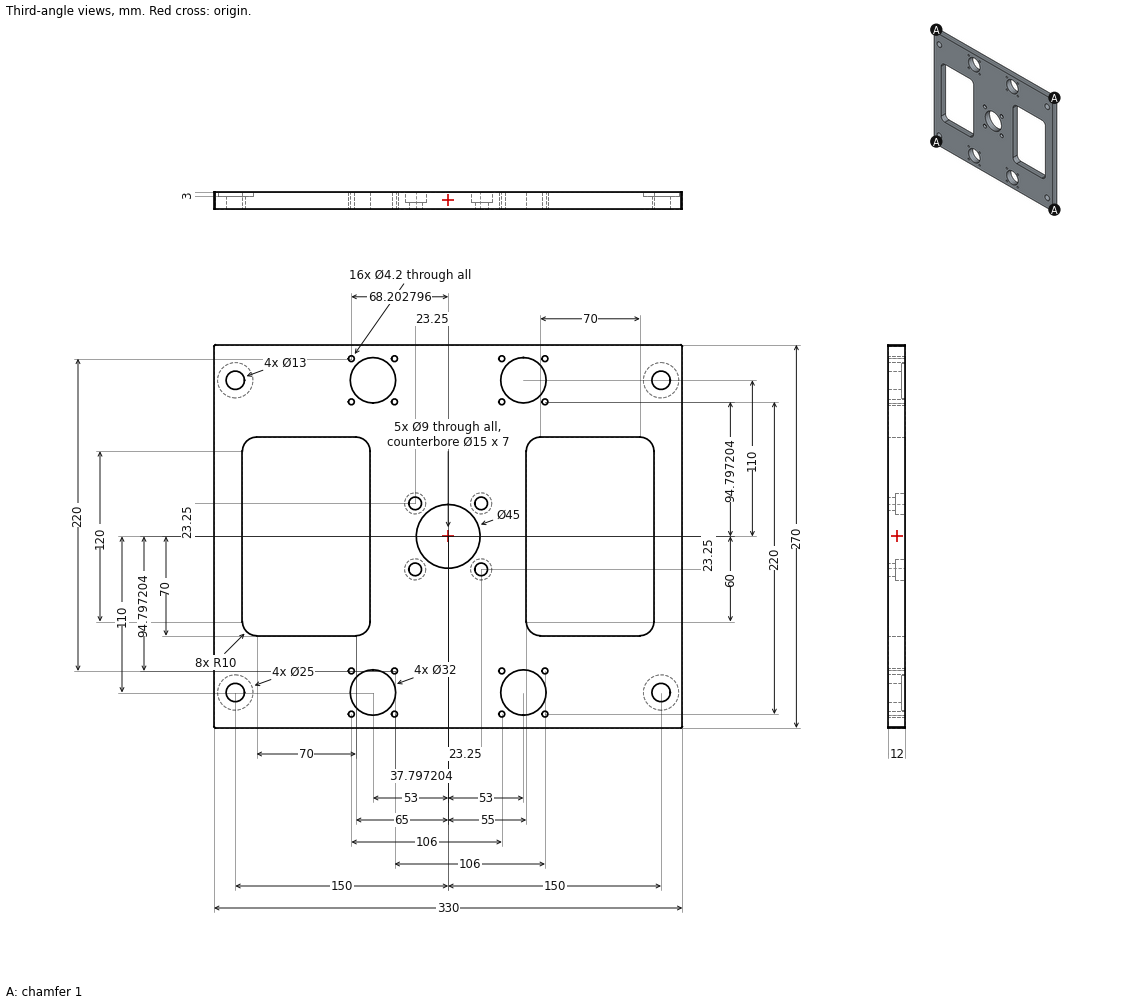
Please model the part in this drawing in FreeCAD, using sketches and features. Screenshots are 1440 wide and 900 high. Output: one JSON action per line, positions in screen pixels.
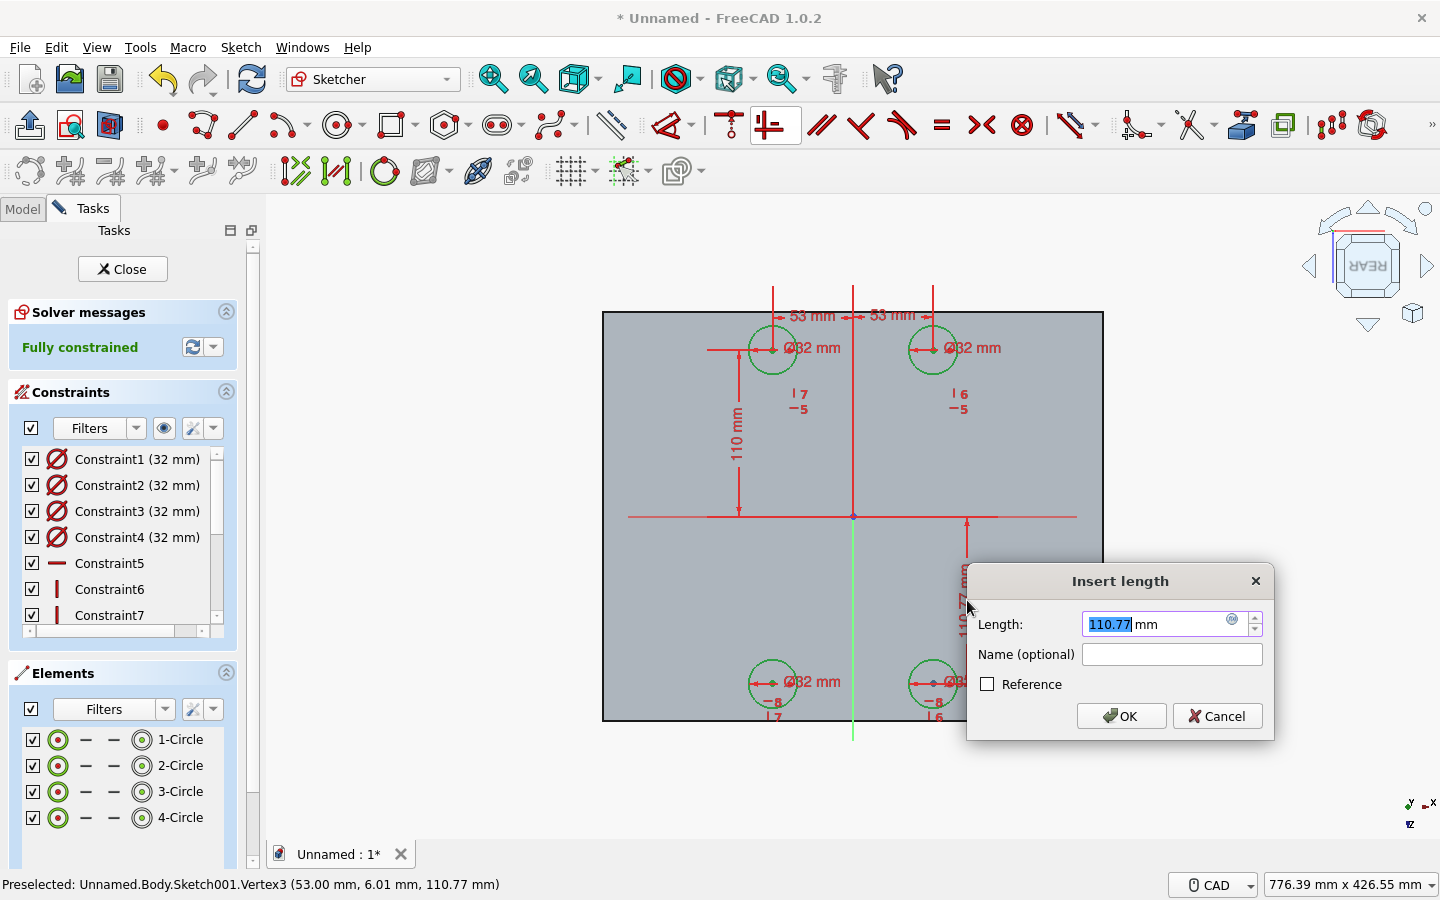
{"action": "type", "text": "110"}
{"action": "key", "text": "Return"}
{"action": "key", "text": "Escape"}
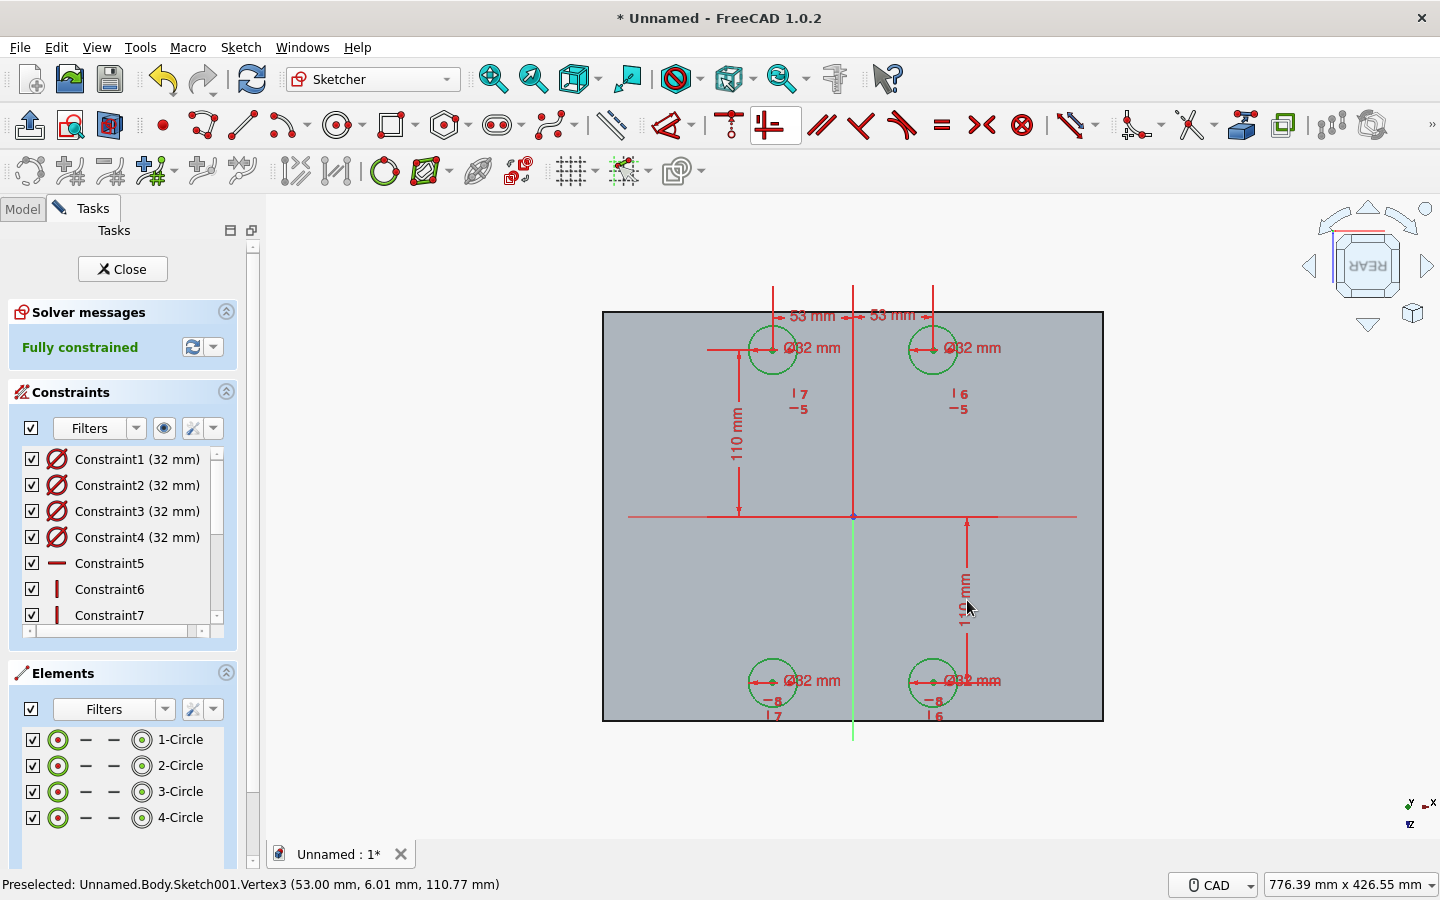
{"action": "left_click", "coordinate": [123, 269]}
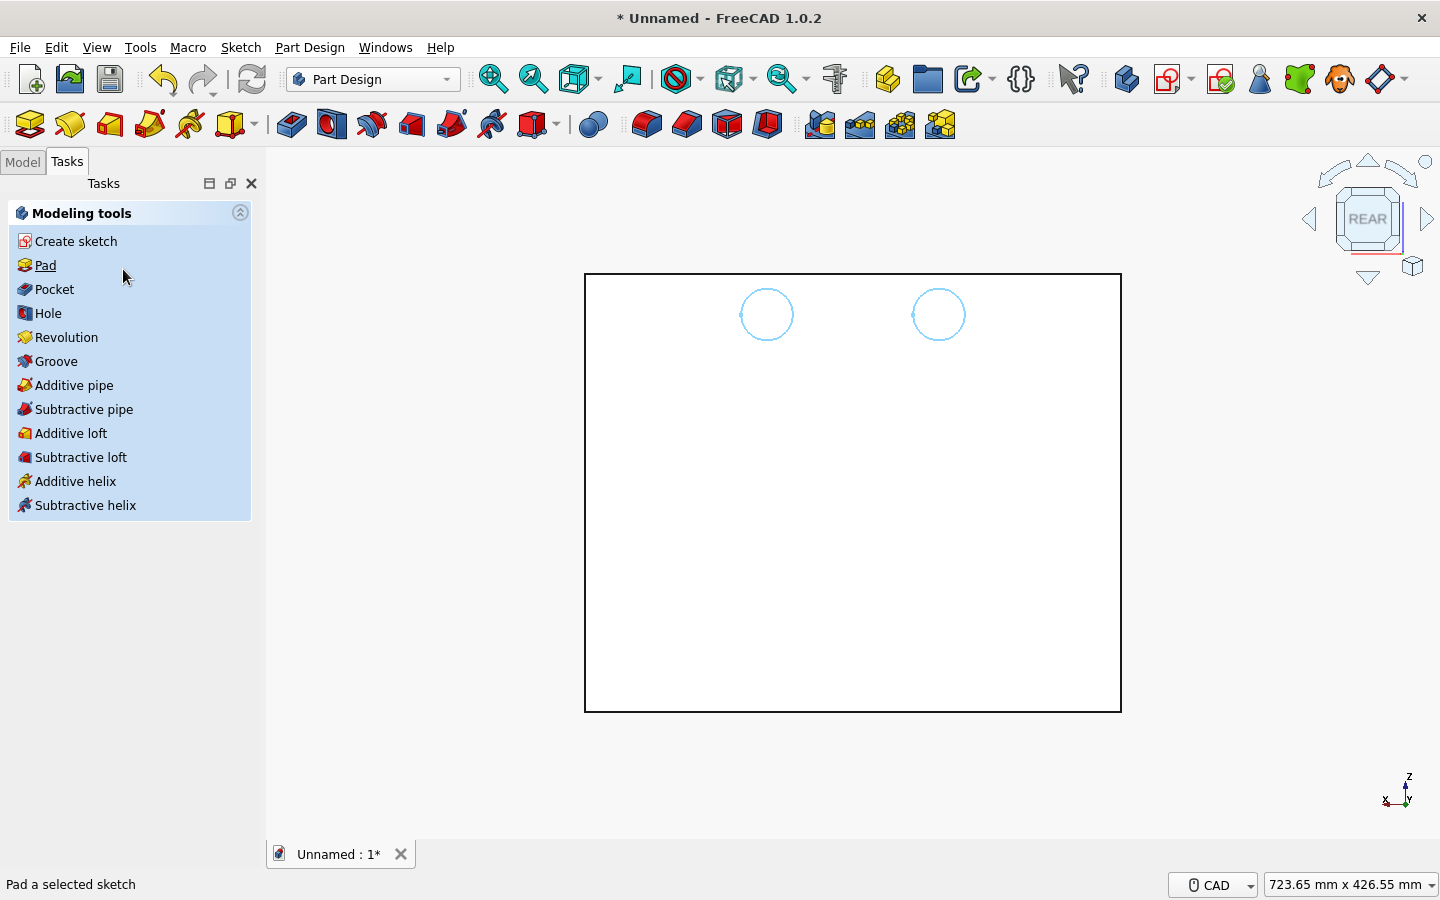
{"action": "left_click", "coordinate": [292, 124]}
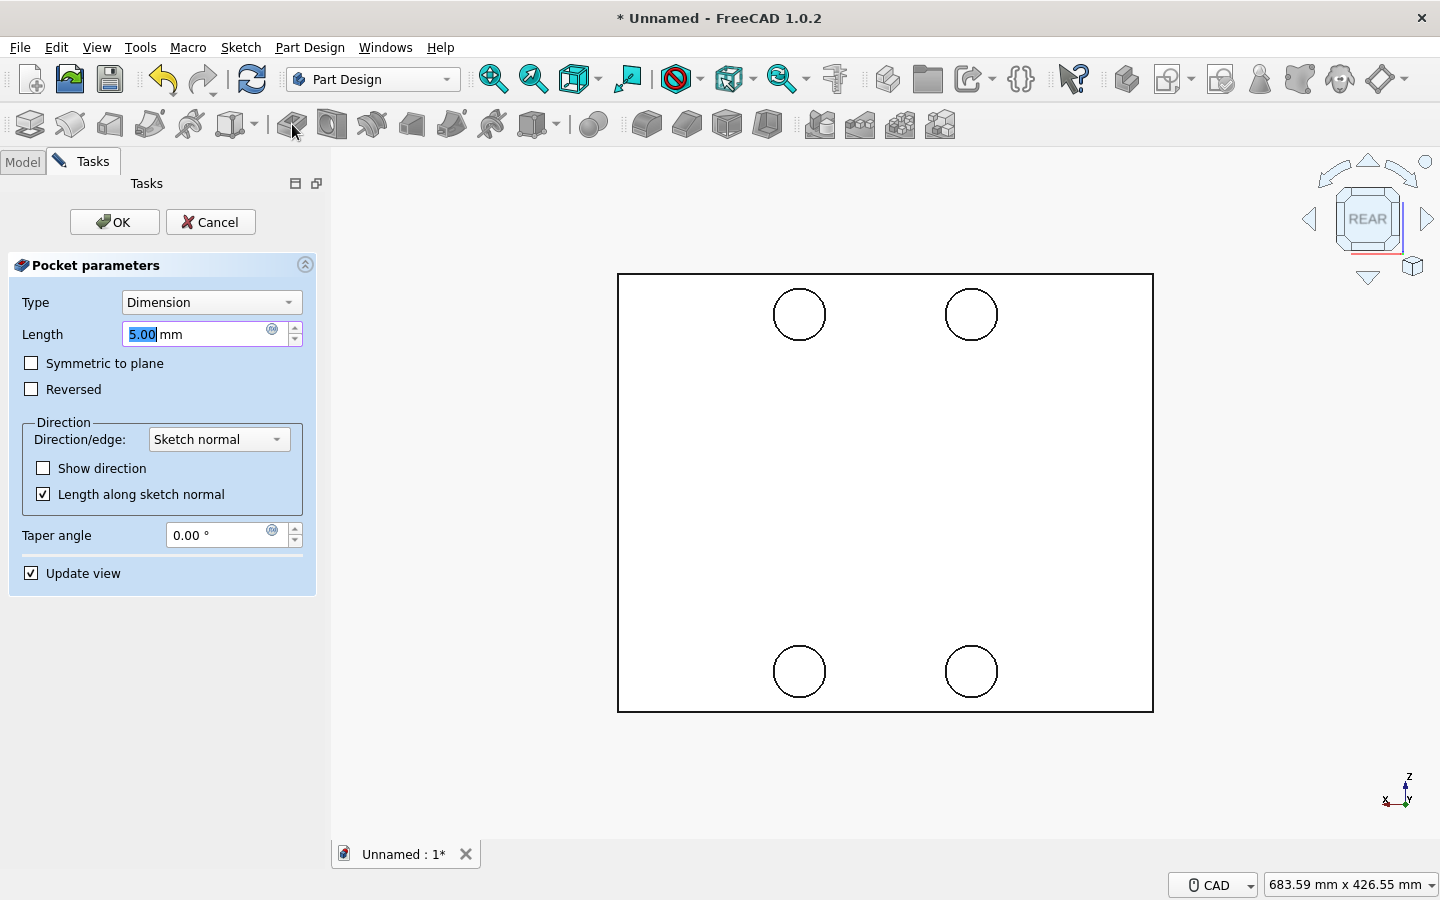
{"action": "left_click", "coordinate": [212, 302]}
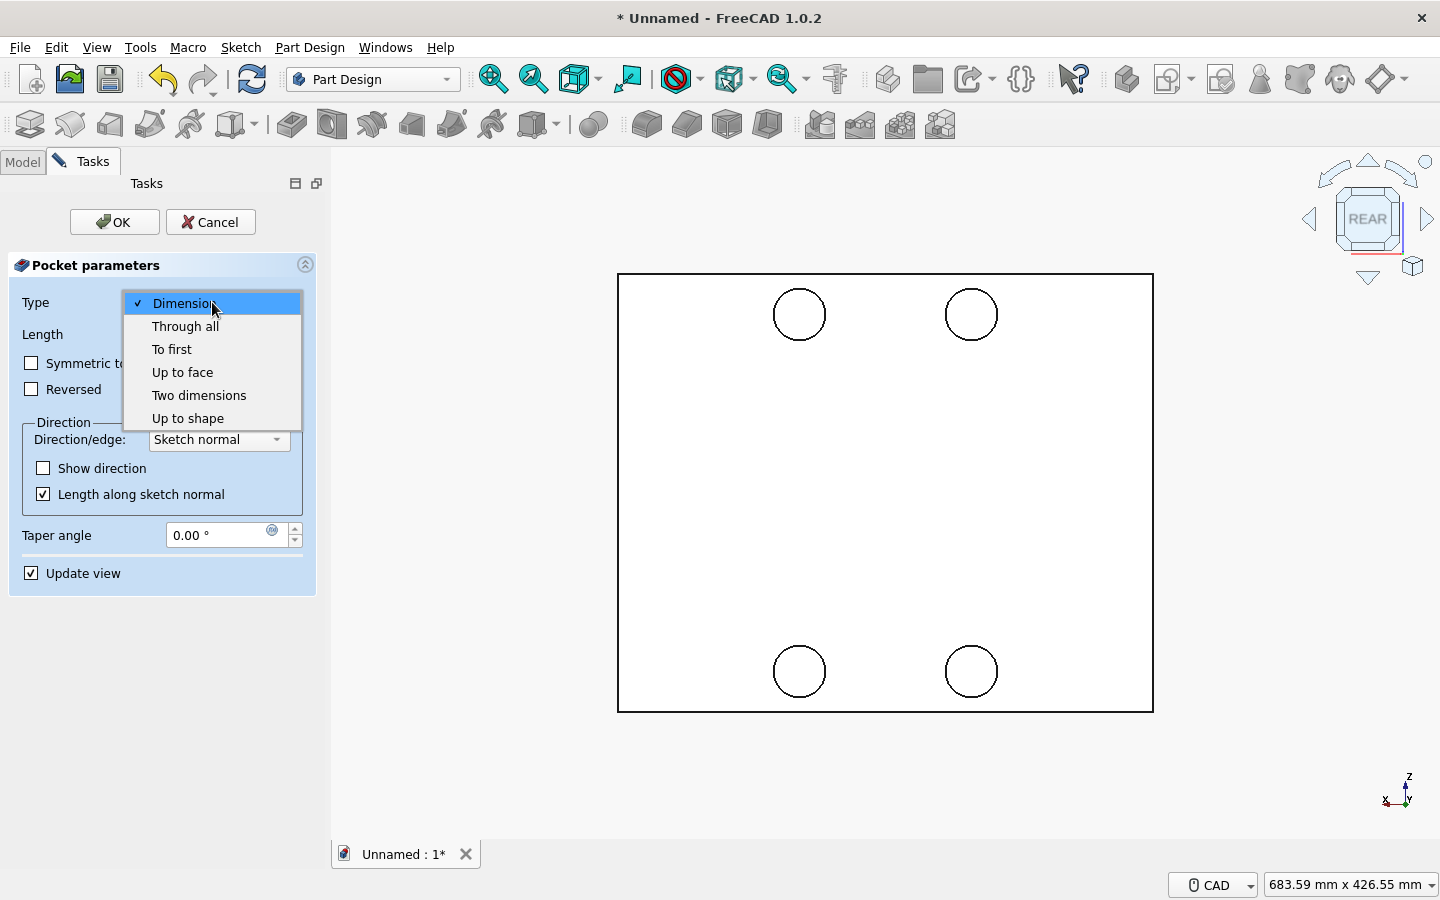
{"action": "left_click", "coordinate": [212, 326]}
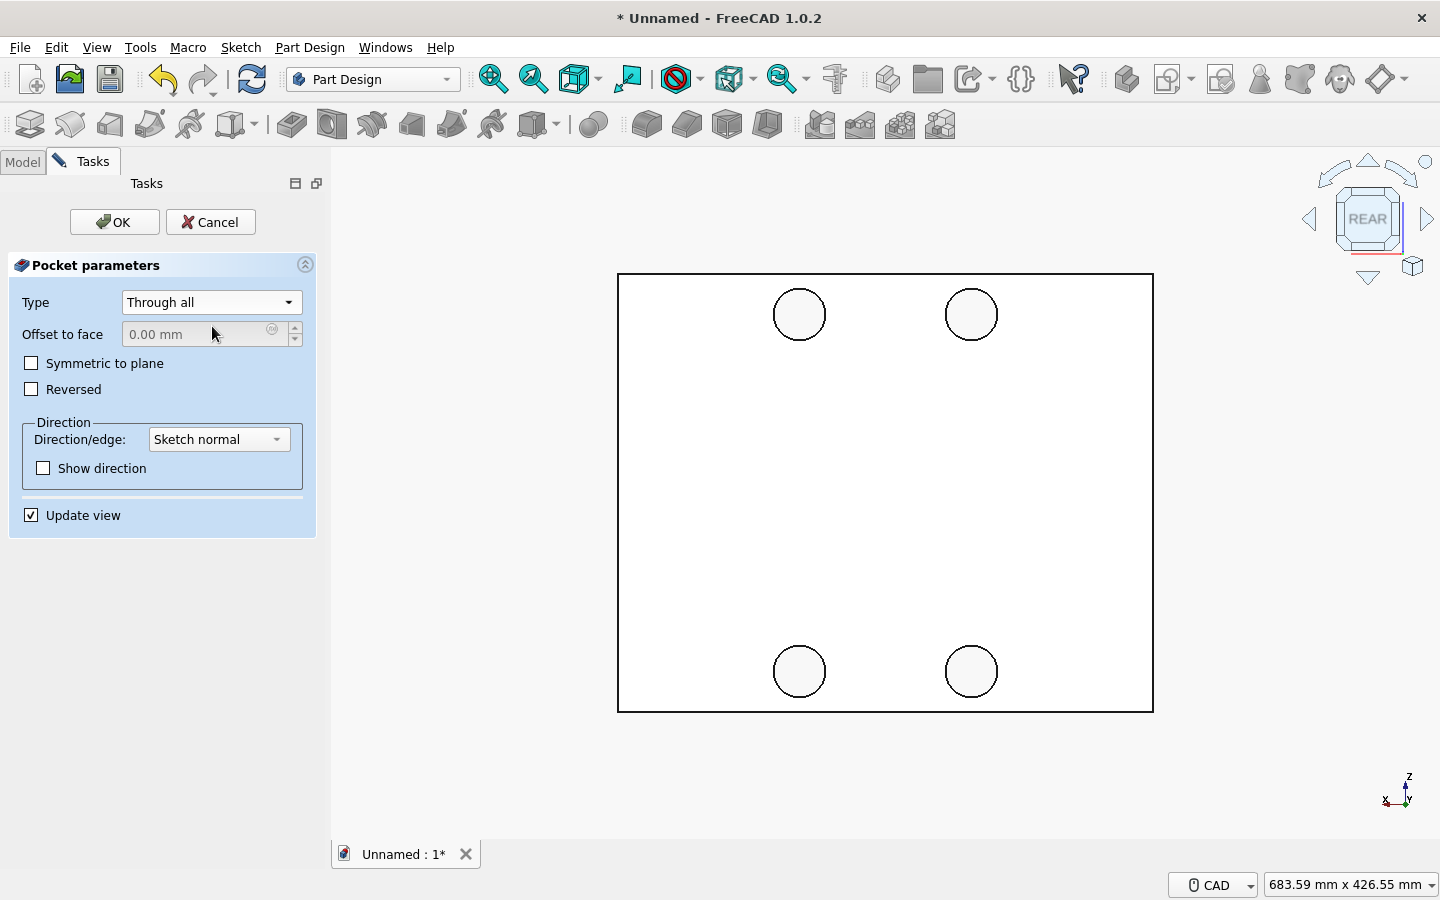
{"action": "left_click", "coordinate": [115, 222]}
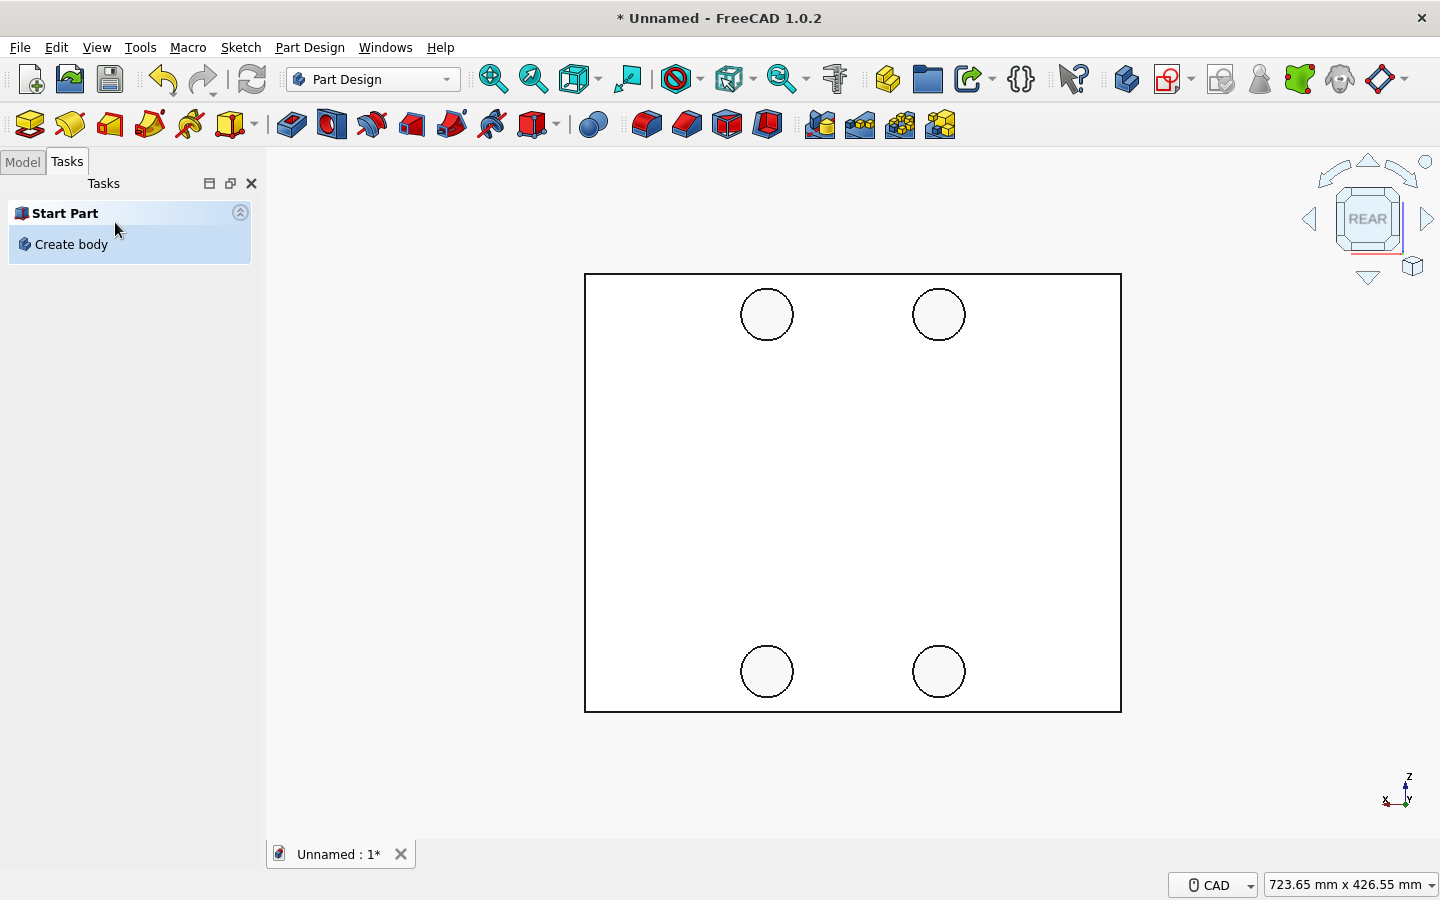
{"action": "left_click", "coordinate": [853, 492]}